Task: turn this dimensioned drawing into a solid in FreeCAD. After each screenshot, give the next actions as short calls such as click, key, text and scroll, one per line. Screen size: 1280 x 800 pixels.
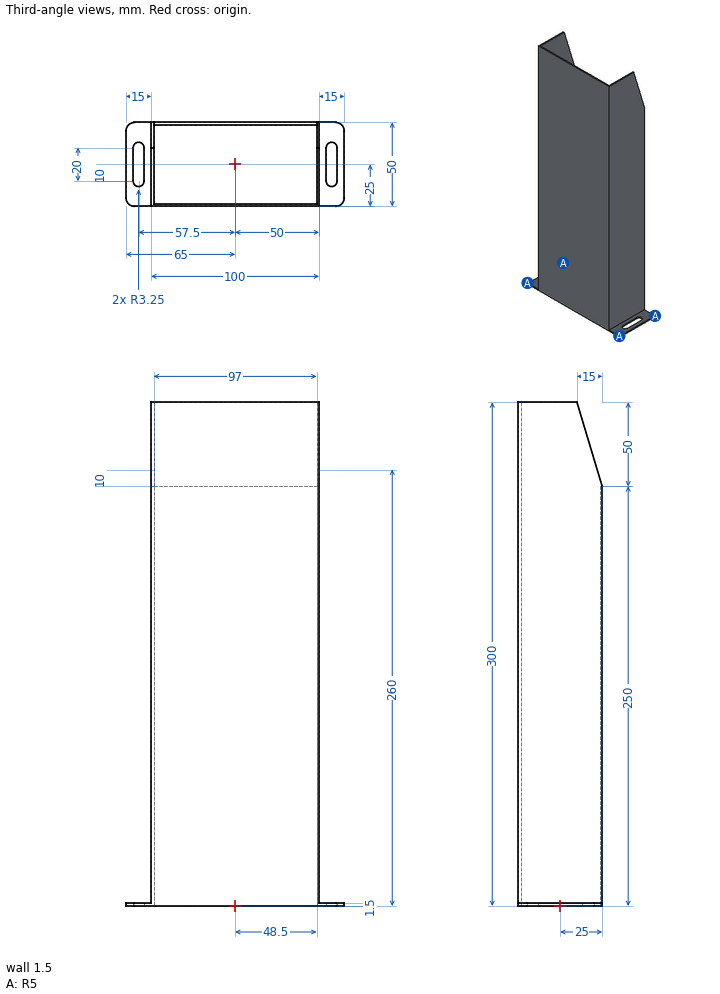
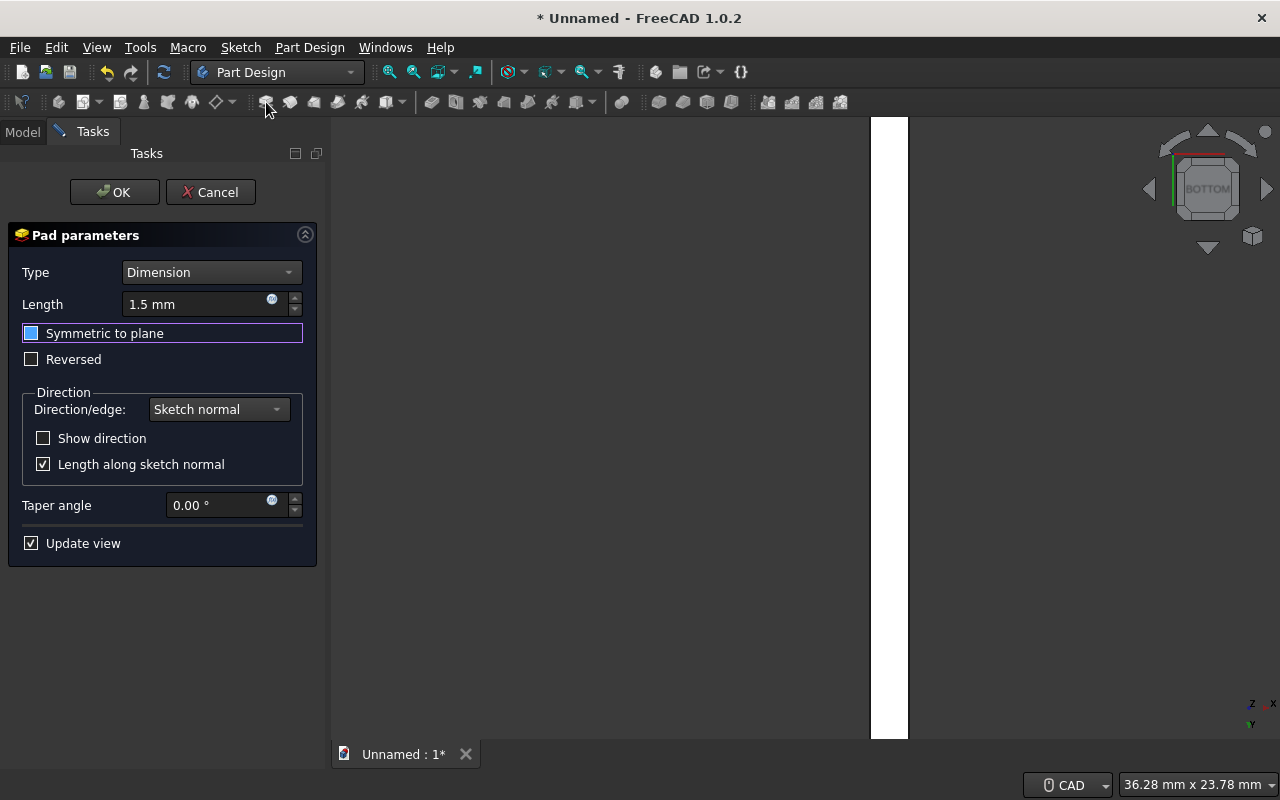
click(30, 359)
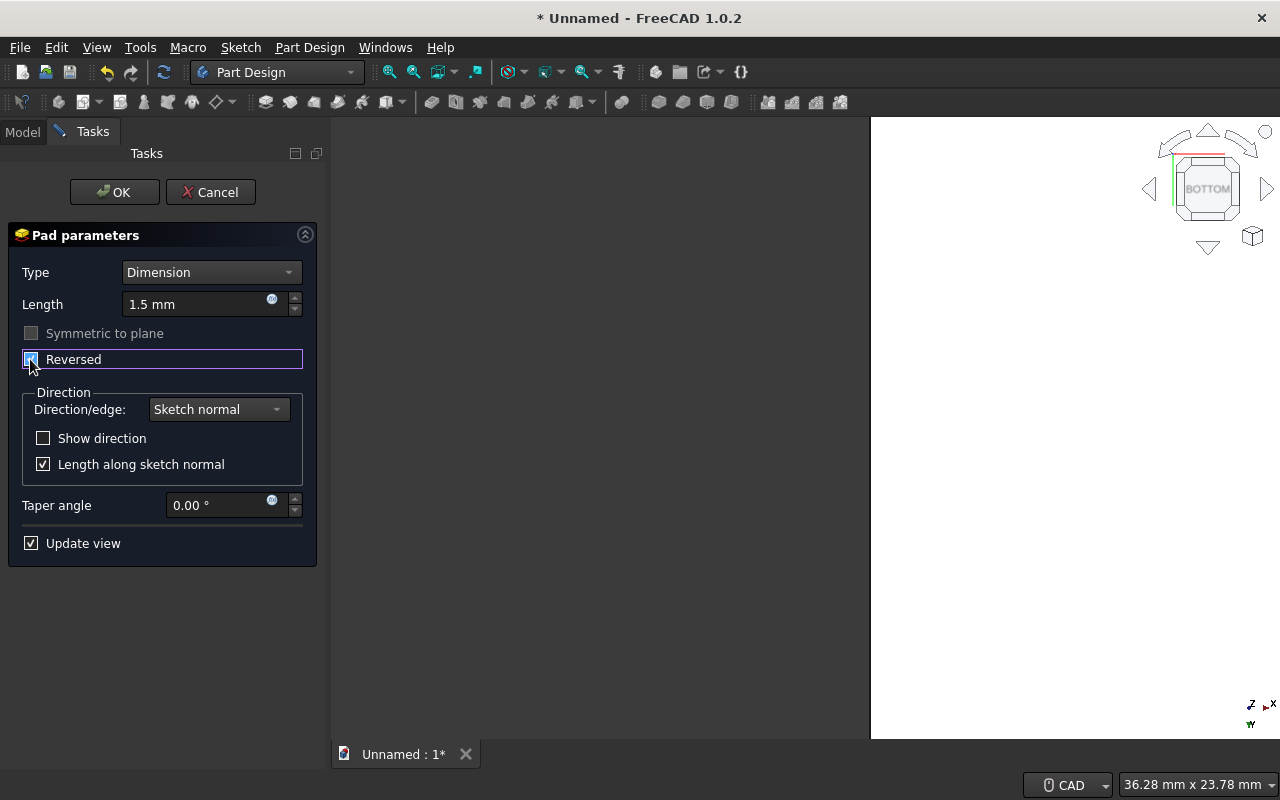
click(115, 192)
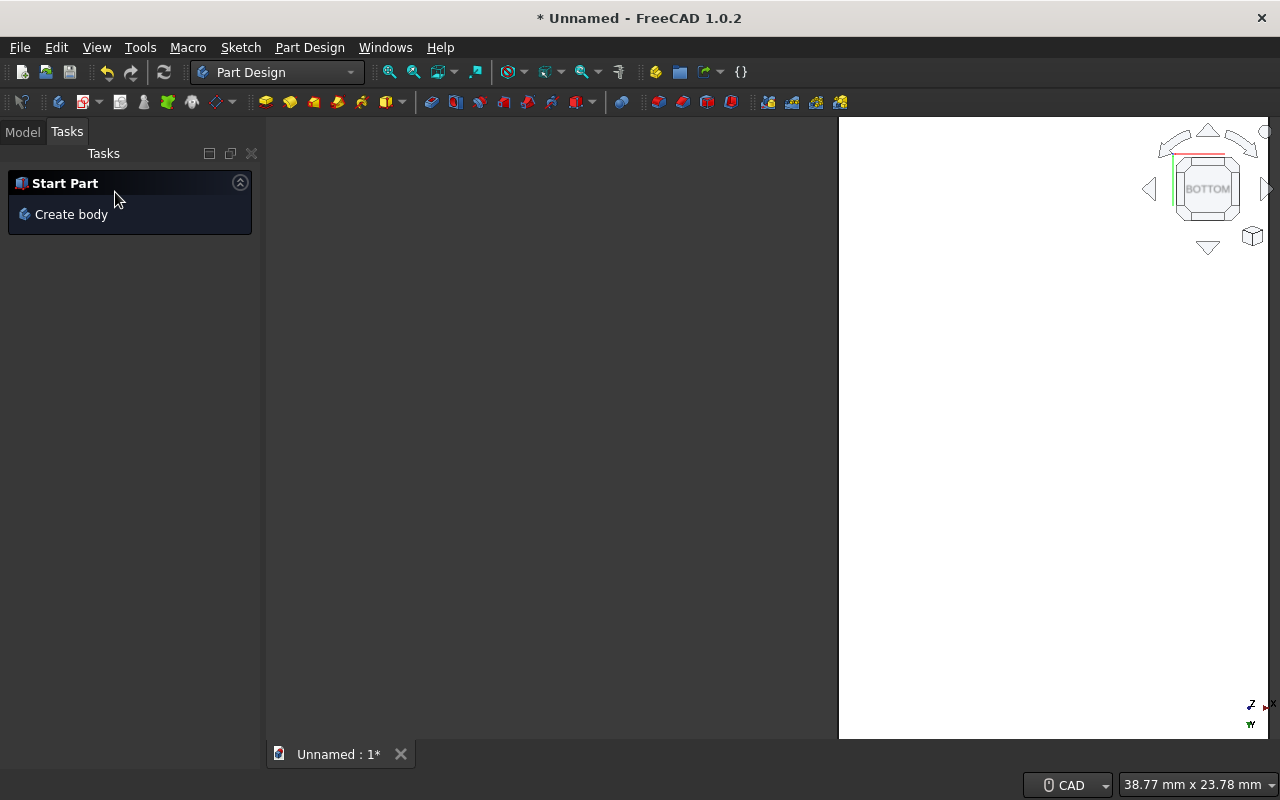
click(390, 72)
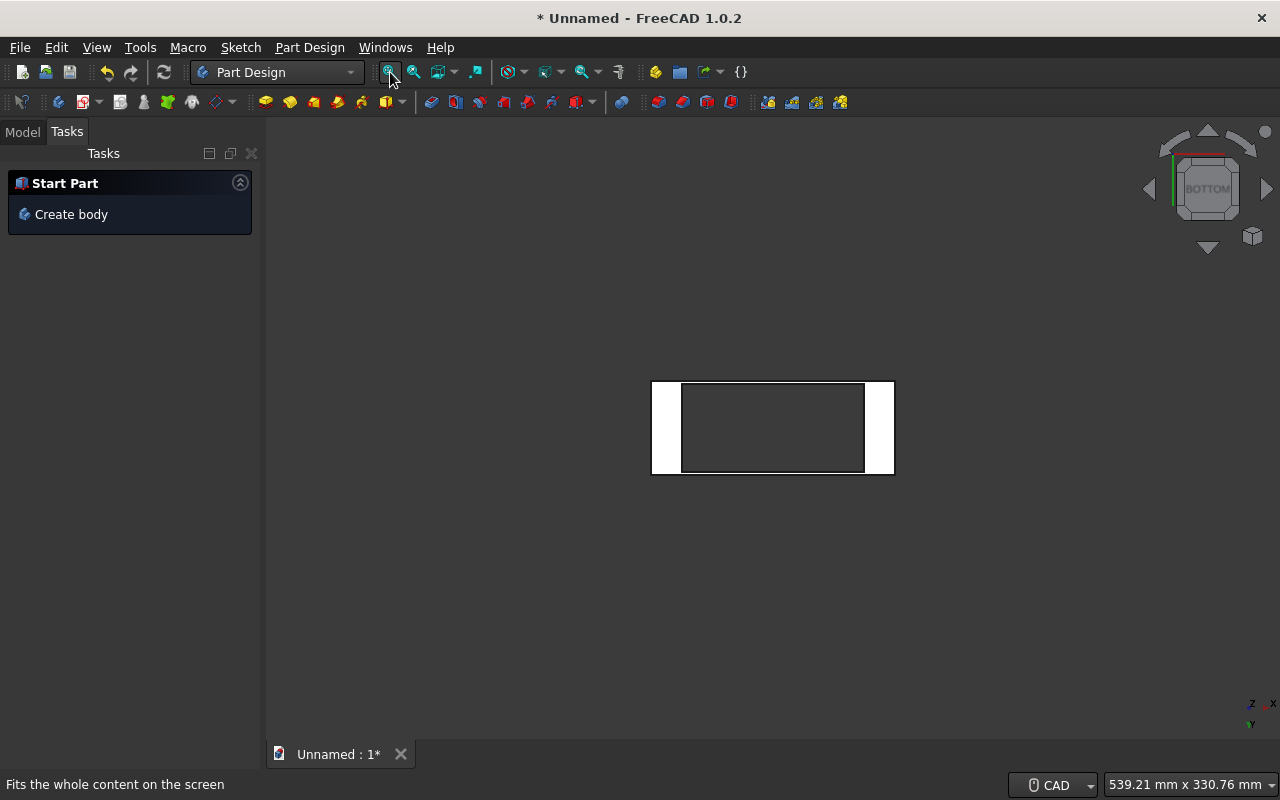
key(0)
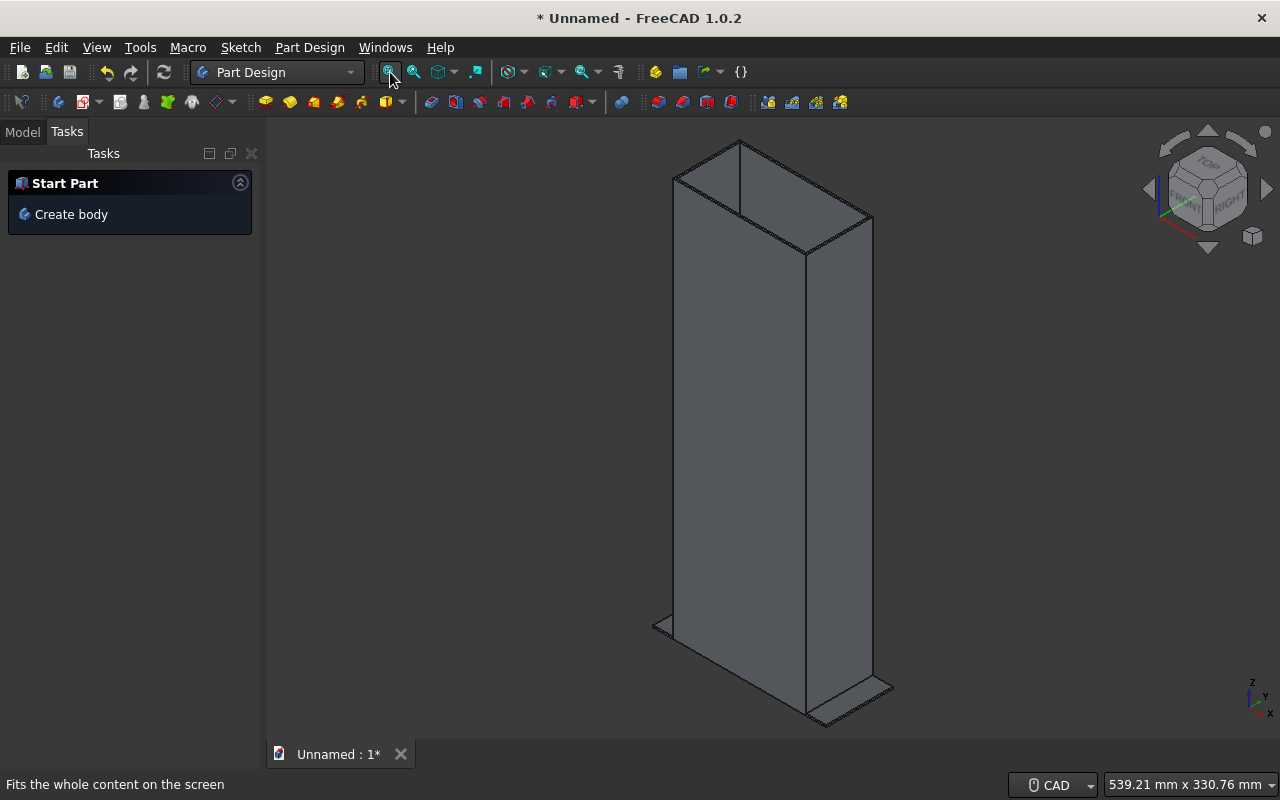
click(839, 333)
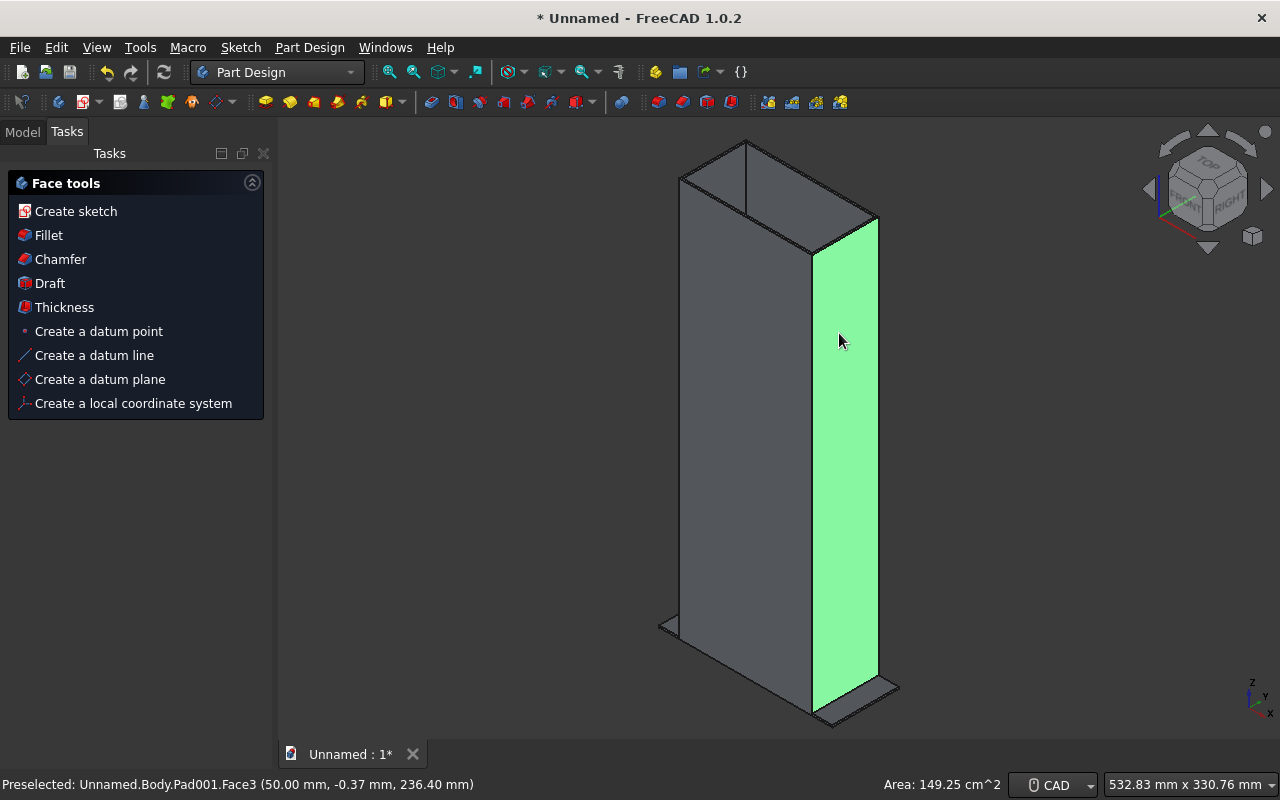
click(84, 102)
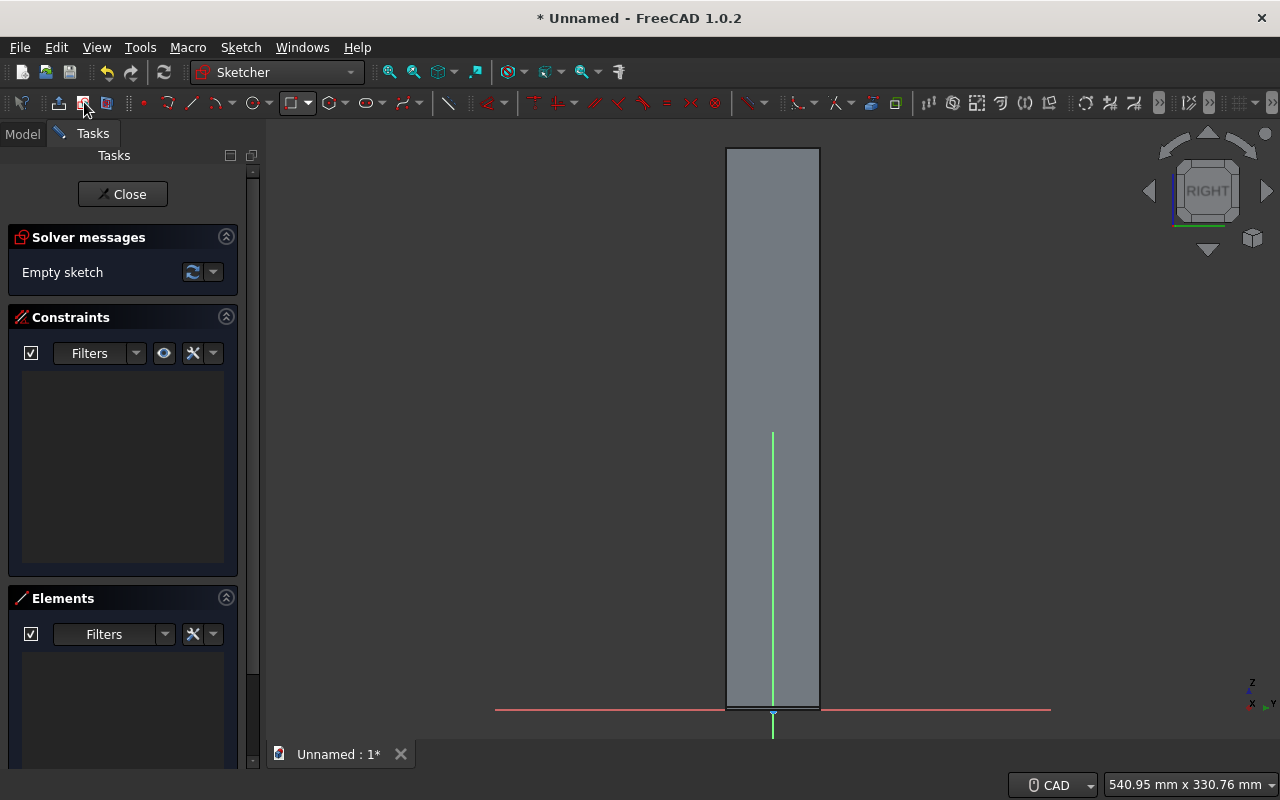
scroll(704, 429, down, 5)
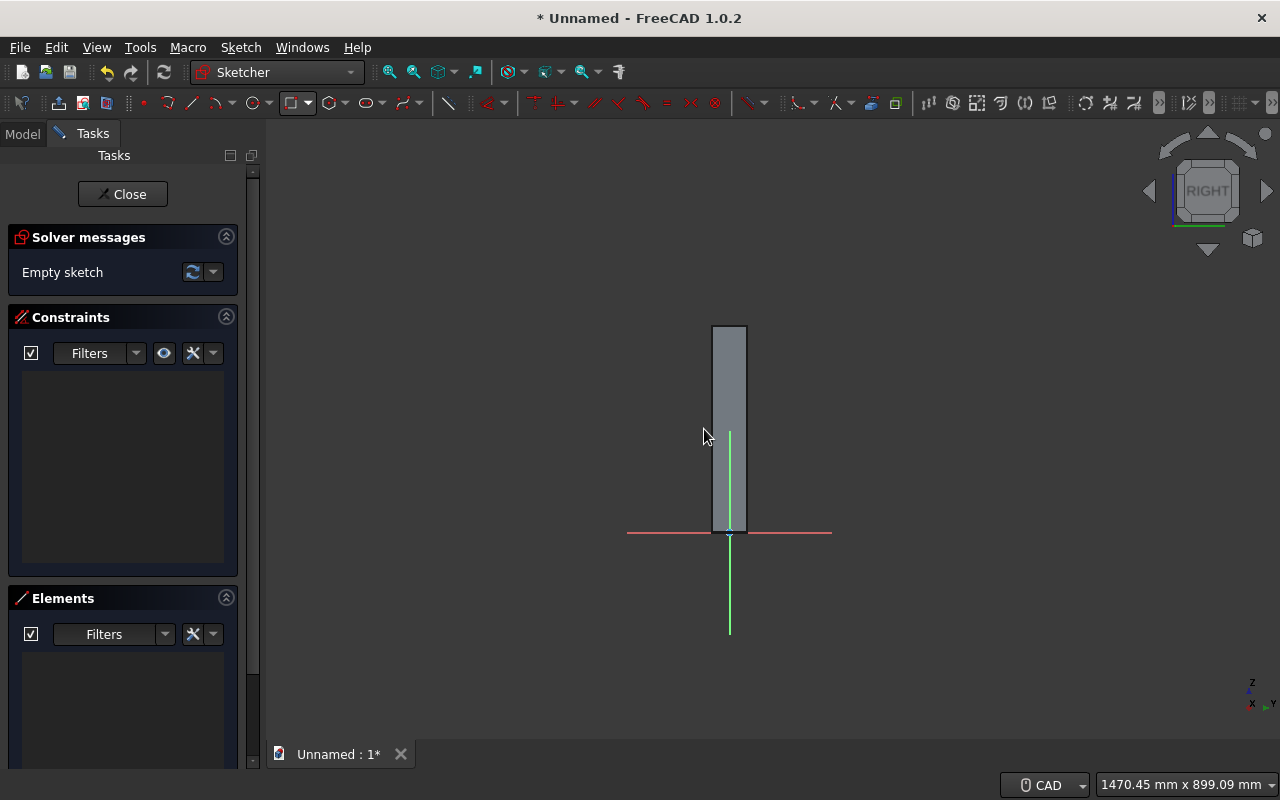
scroll(745, 335, up, 12)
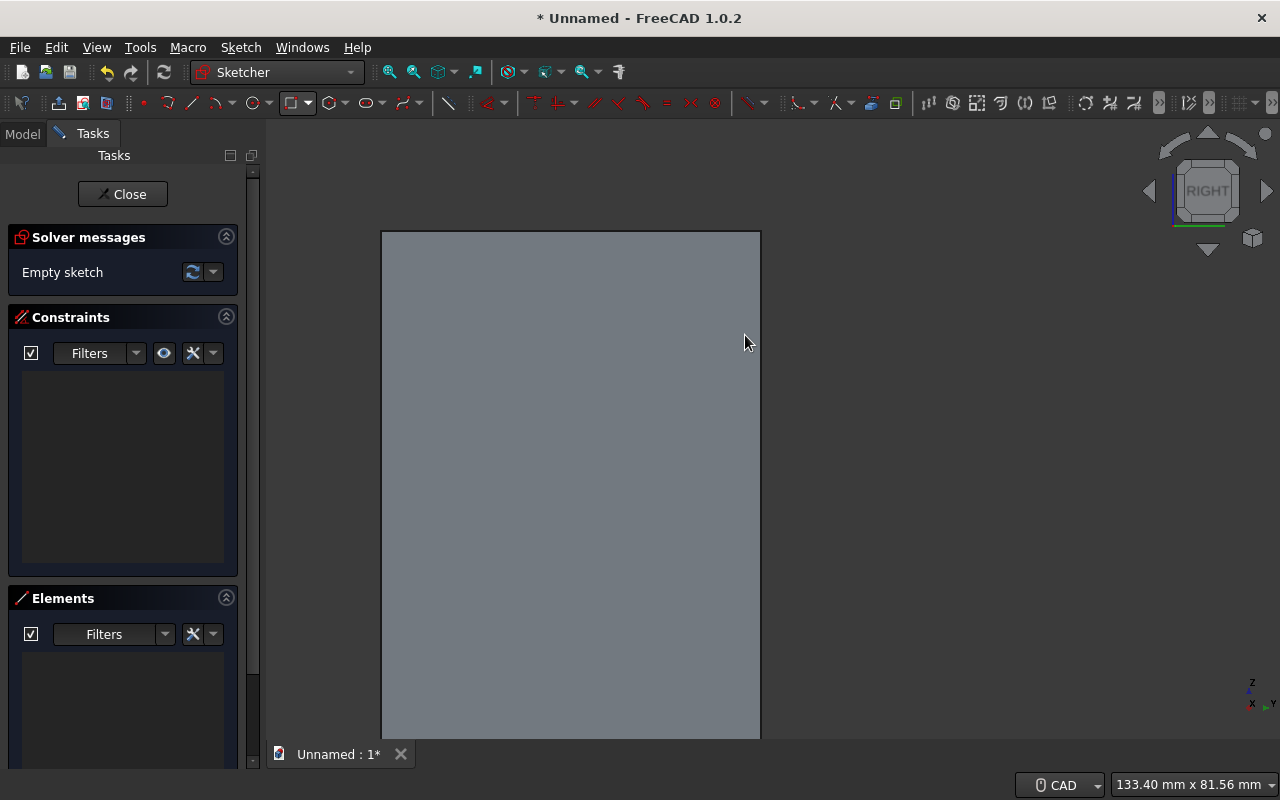
click(168, 104)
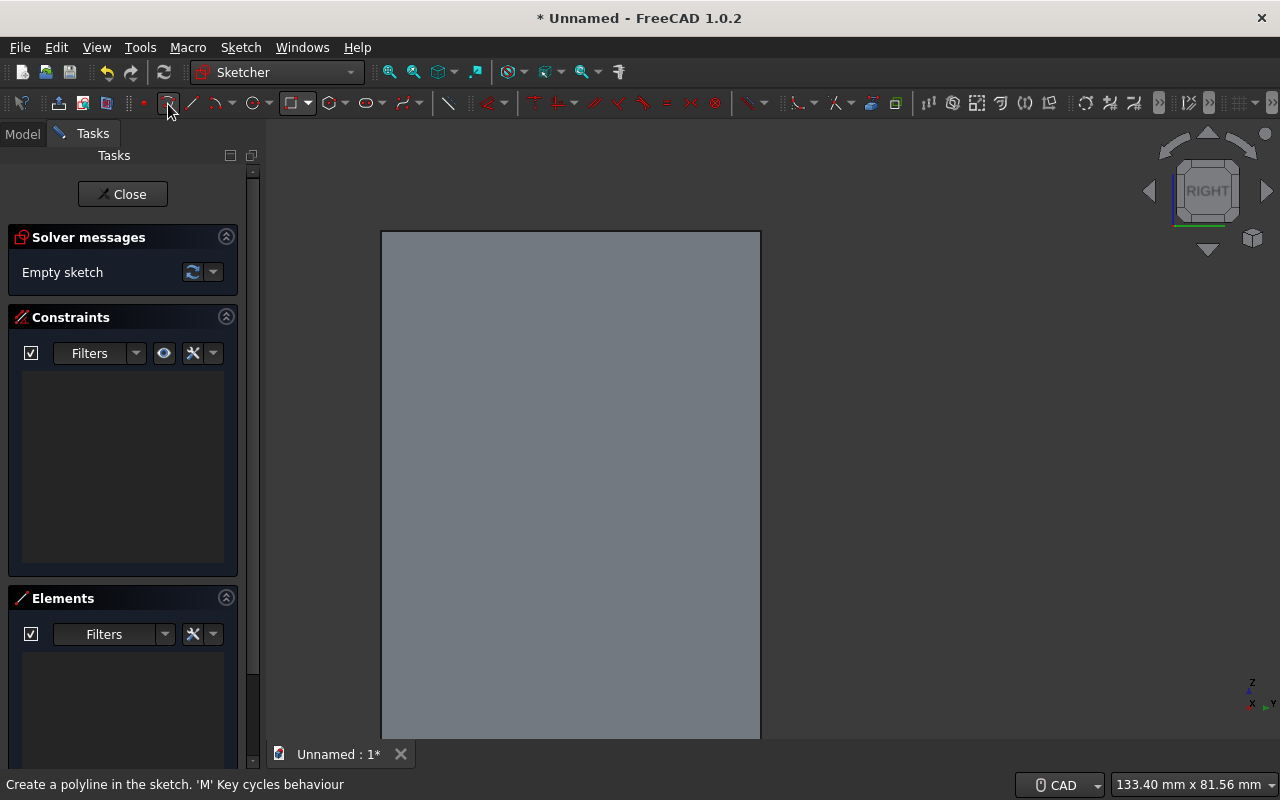
click(761, 611)
click(761, 231)
click(647, 231)
click(761, 612)
key(Escape)
key(Escape)